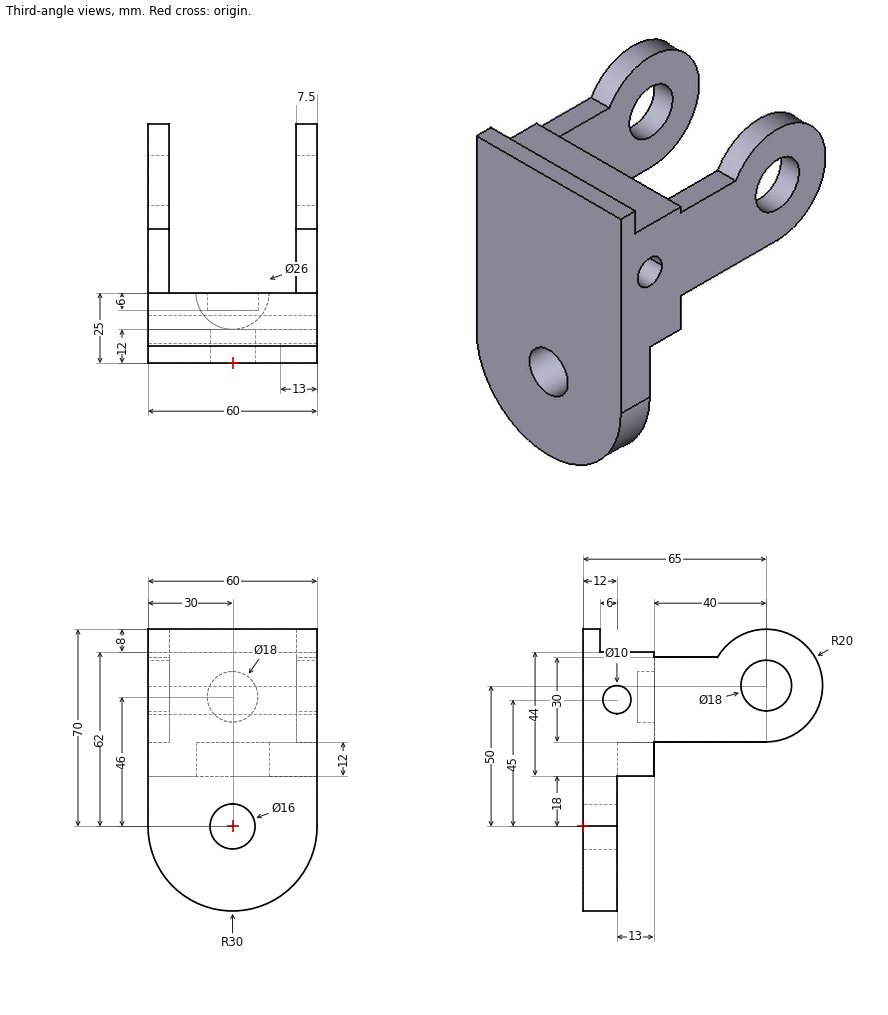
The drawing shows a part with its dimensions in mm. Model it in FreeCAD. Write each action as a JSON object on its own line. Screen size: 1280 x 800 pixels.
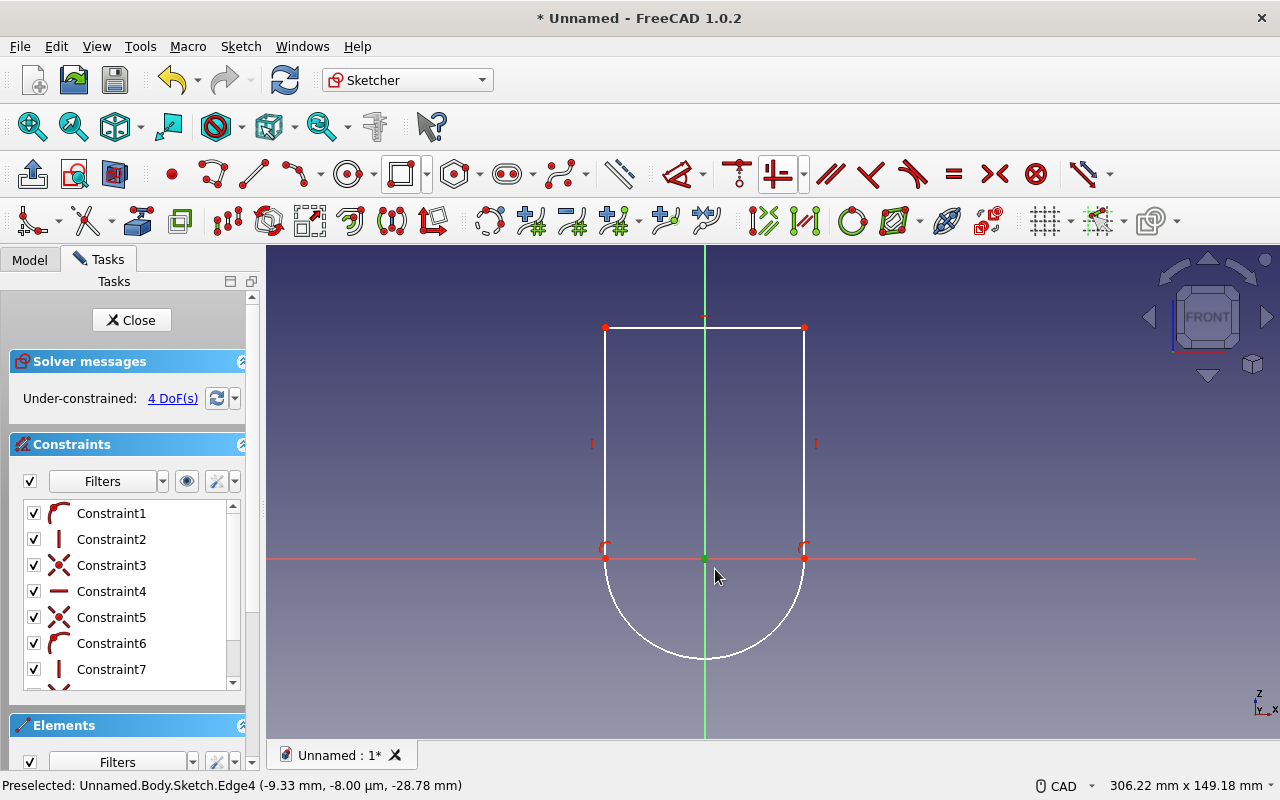
{"action": "left_click", "coordinate": [737, 174]}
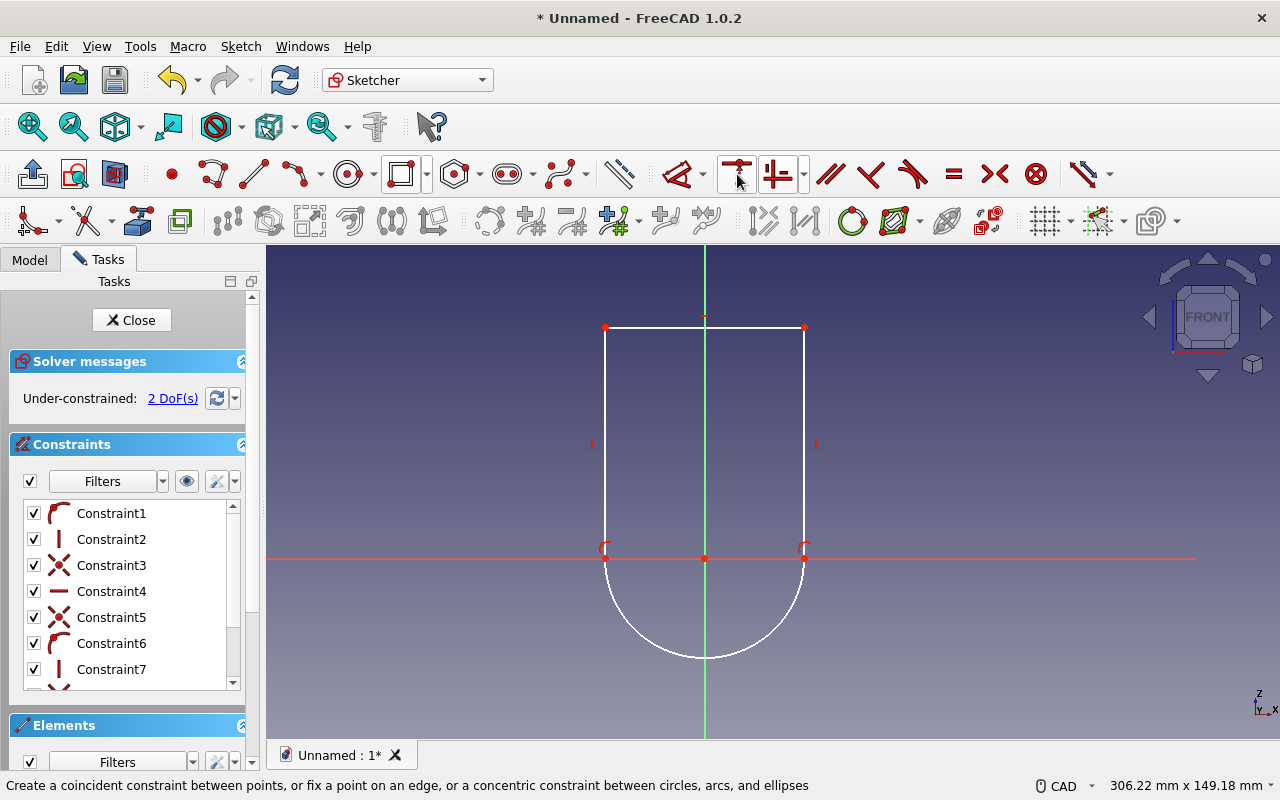
{"action": "key", "text": "d"}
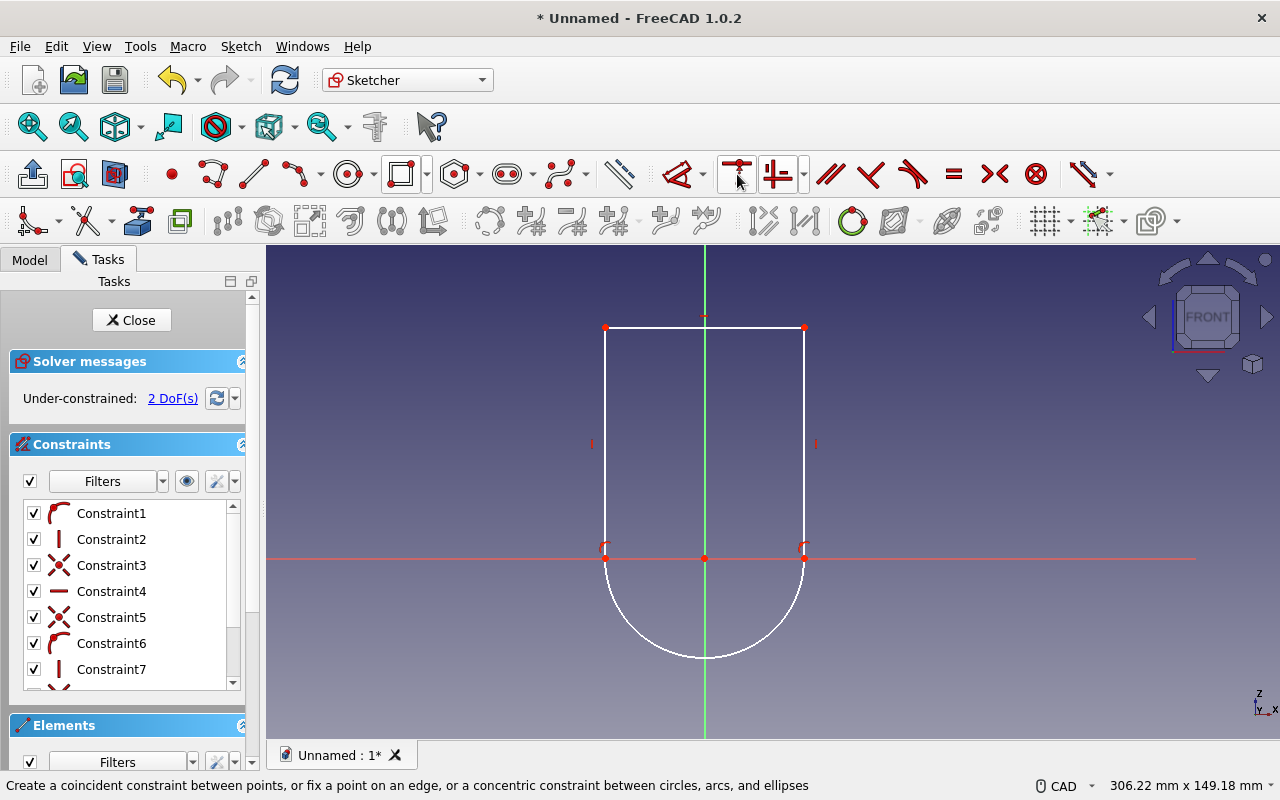
{"action": "left_click", "coordinate": [646, 639]}
{"action": "left_click", "coordinate": [627, 665]}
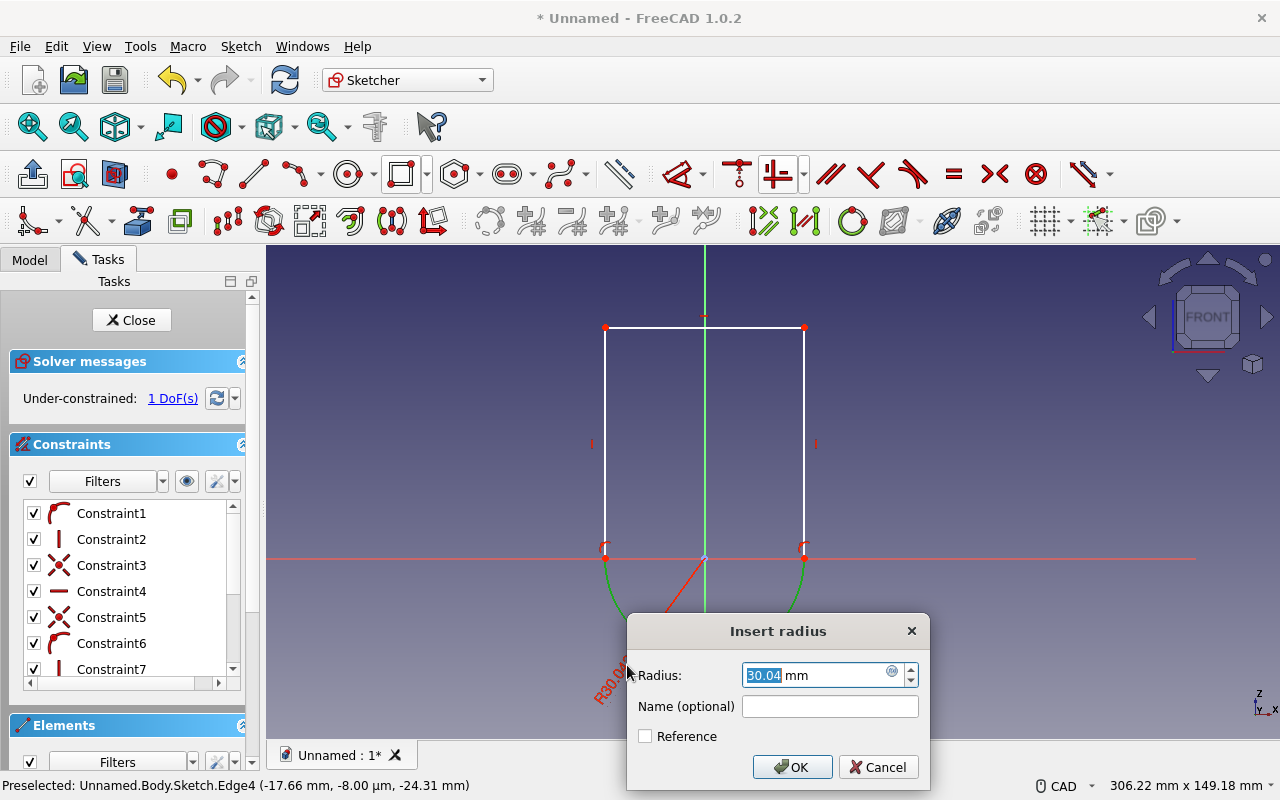
{"action": "type", "text": "30"}
{"action": "key", "text": "Return"}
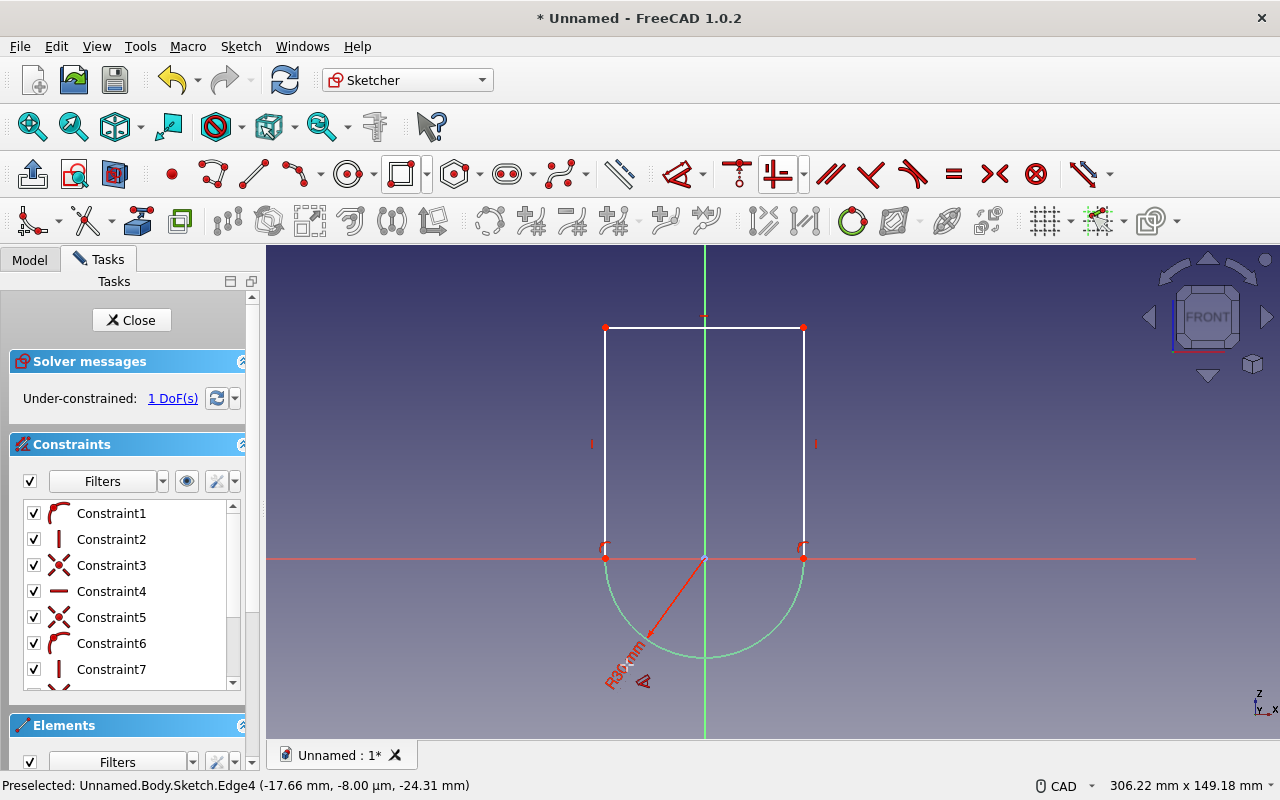
{"action": "left_click", "coordinate": [605, 489]}
{"action": "left_click", "coordinate": [571, 443]}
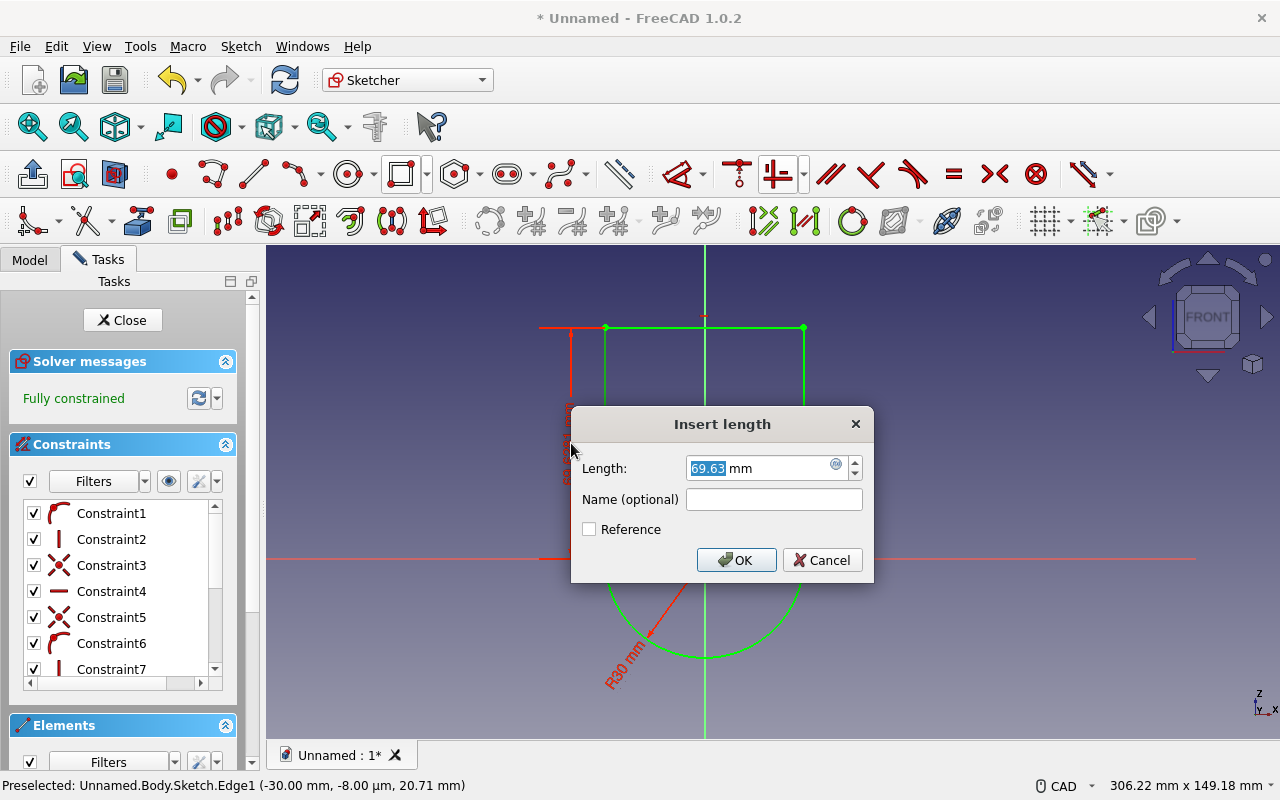
{"action": "type", "text": "70"}
{"action": "key", "text": "Return"}
{"action": "key", "text": "Escape"}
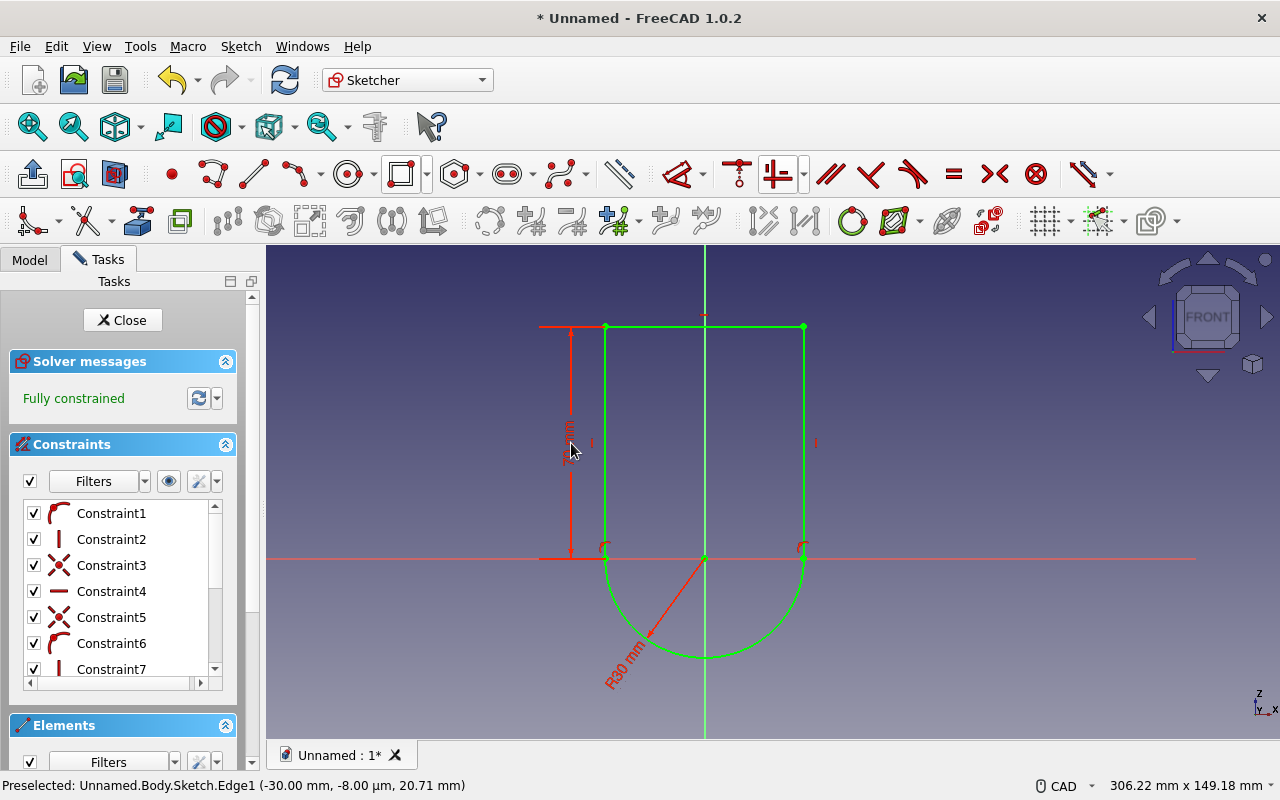
{"action": "left_click", "coordinate": [123, 320]}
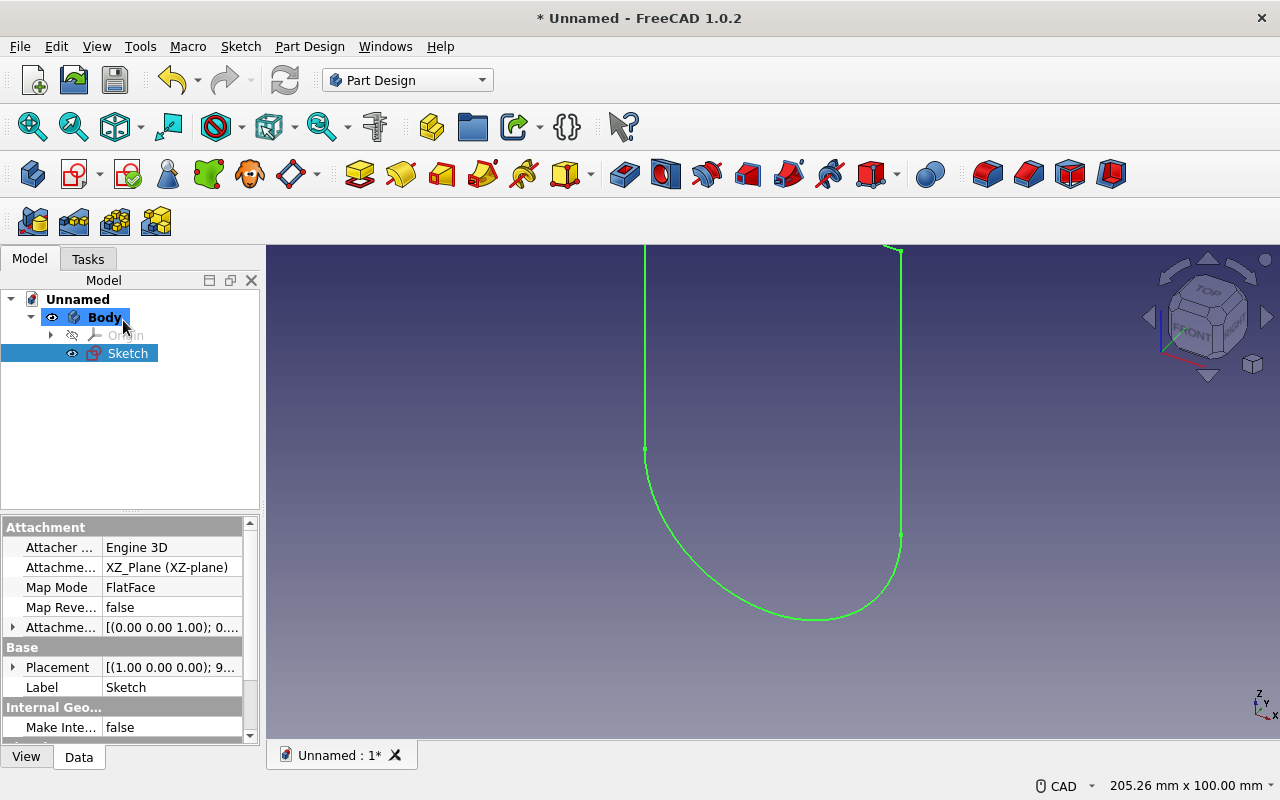
{"action": "left_click", "coordinate": [360, 174]}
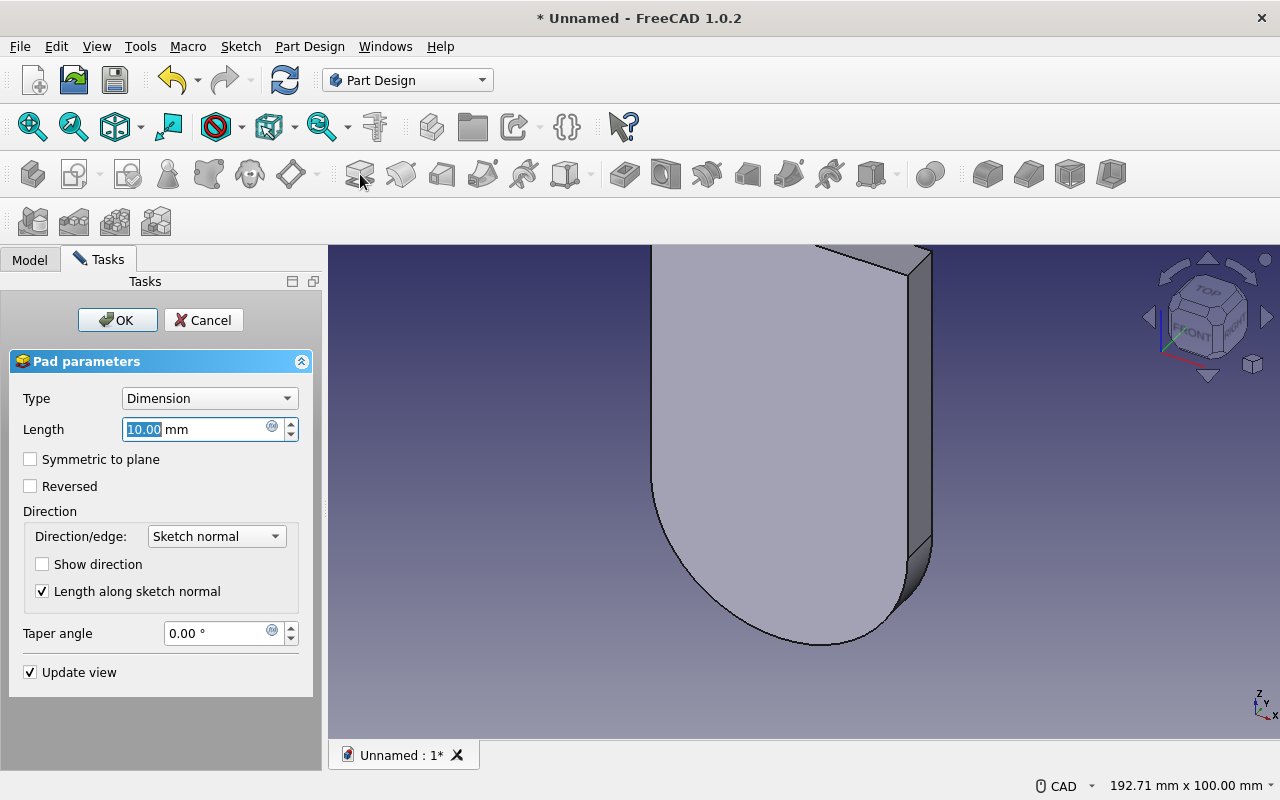
{"action": "type", "text": "12"}
{"action": "key", "text": "Tab"}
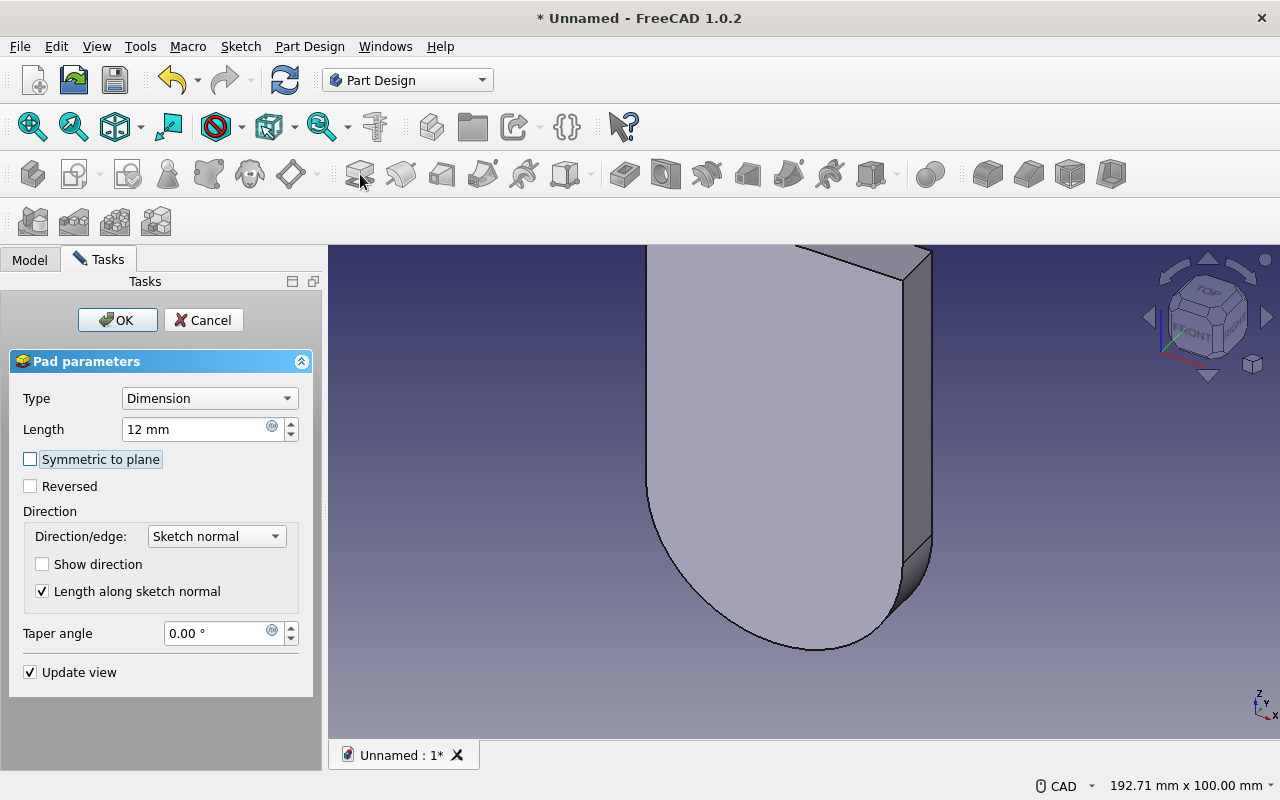
{"action": "left_click", "coordinate": [31, 486]}